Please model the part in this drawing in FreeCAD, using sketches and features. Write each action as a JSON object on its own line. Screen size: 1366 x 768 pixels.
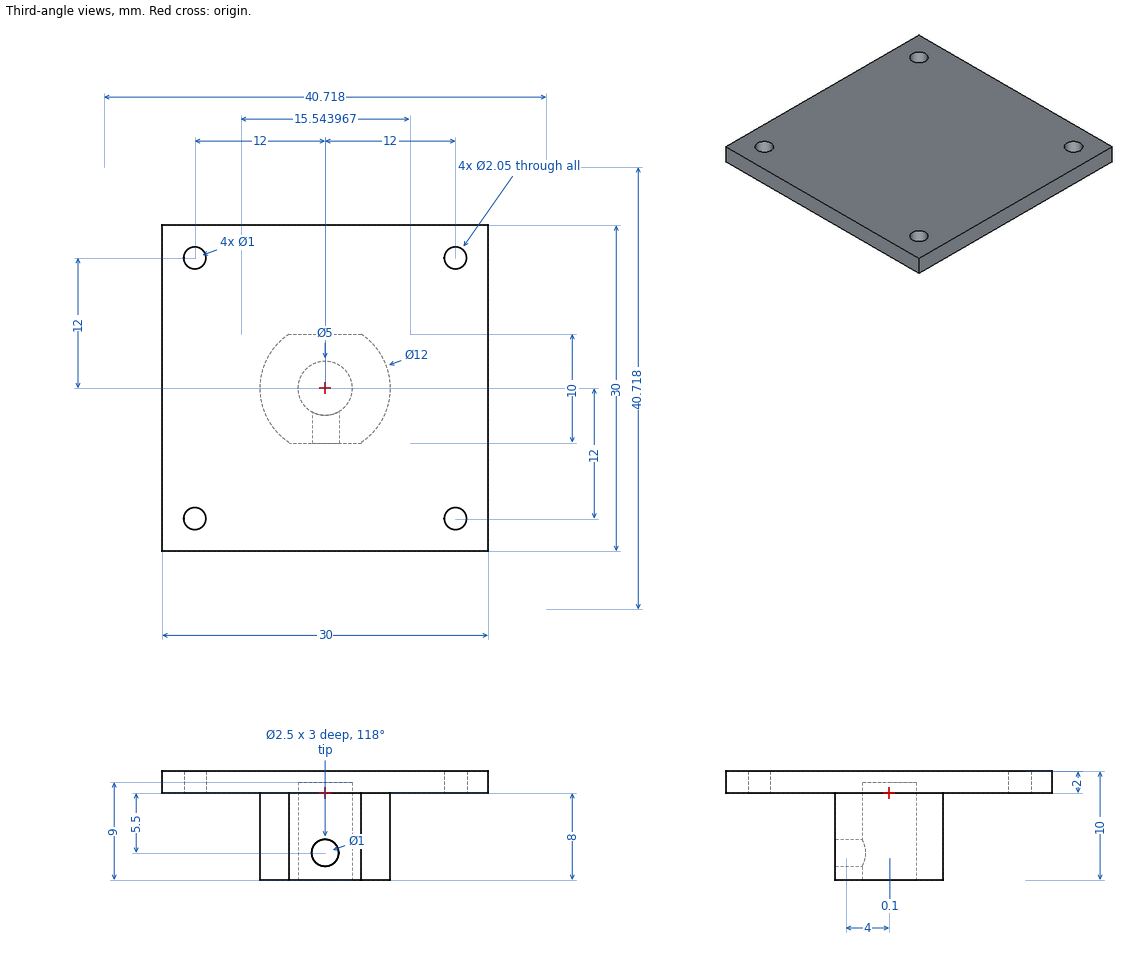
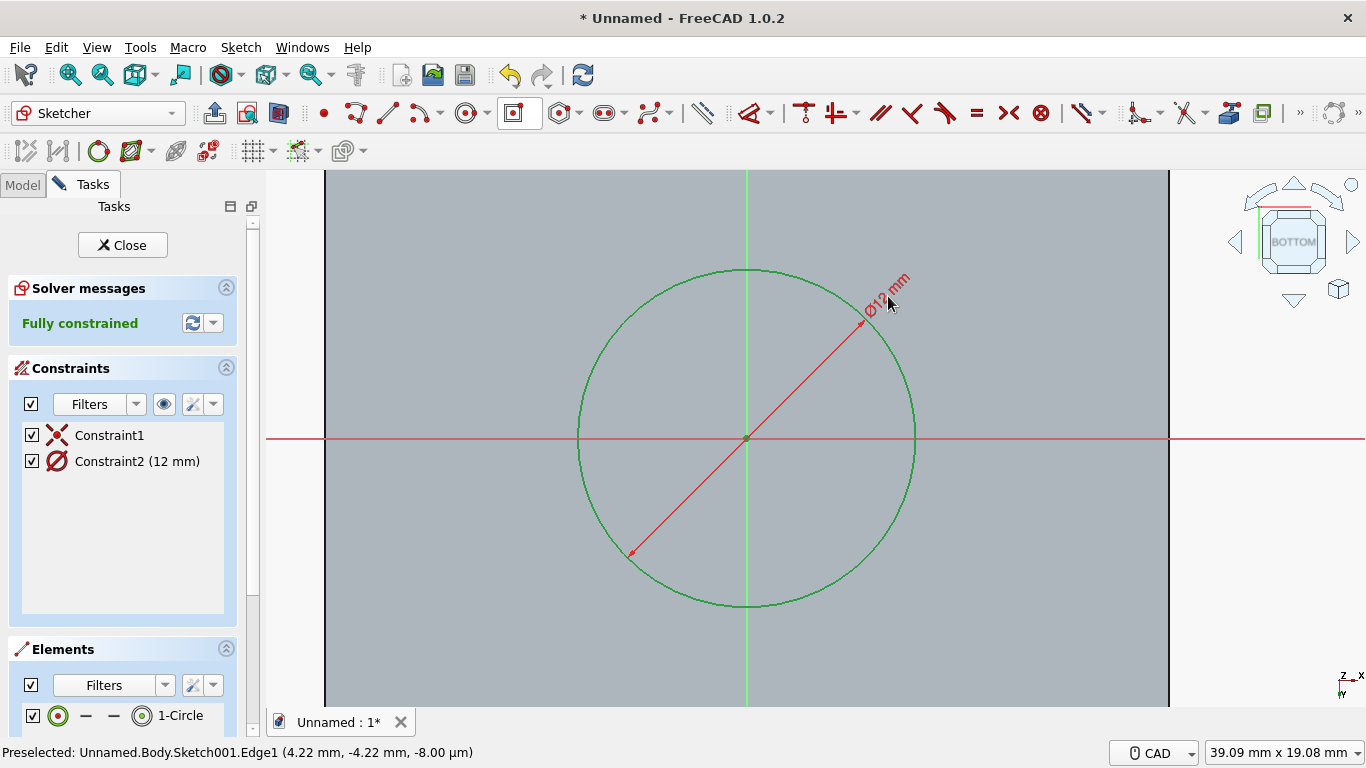
{"action": "left_click", "coordinate": [123, 245]}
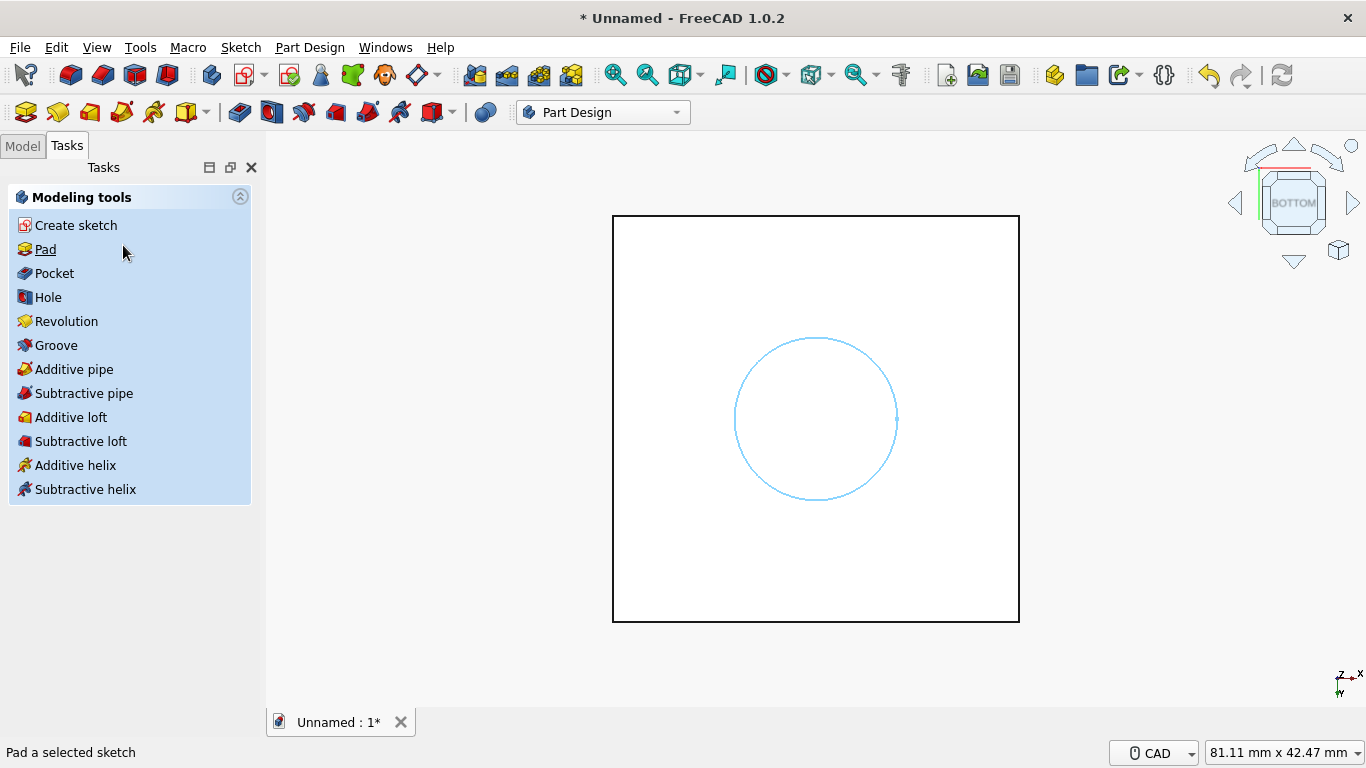
{"action": "left_click", "coordinate": [26, 112]}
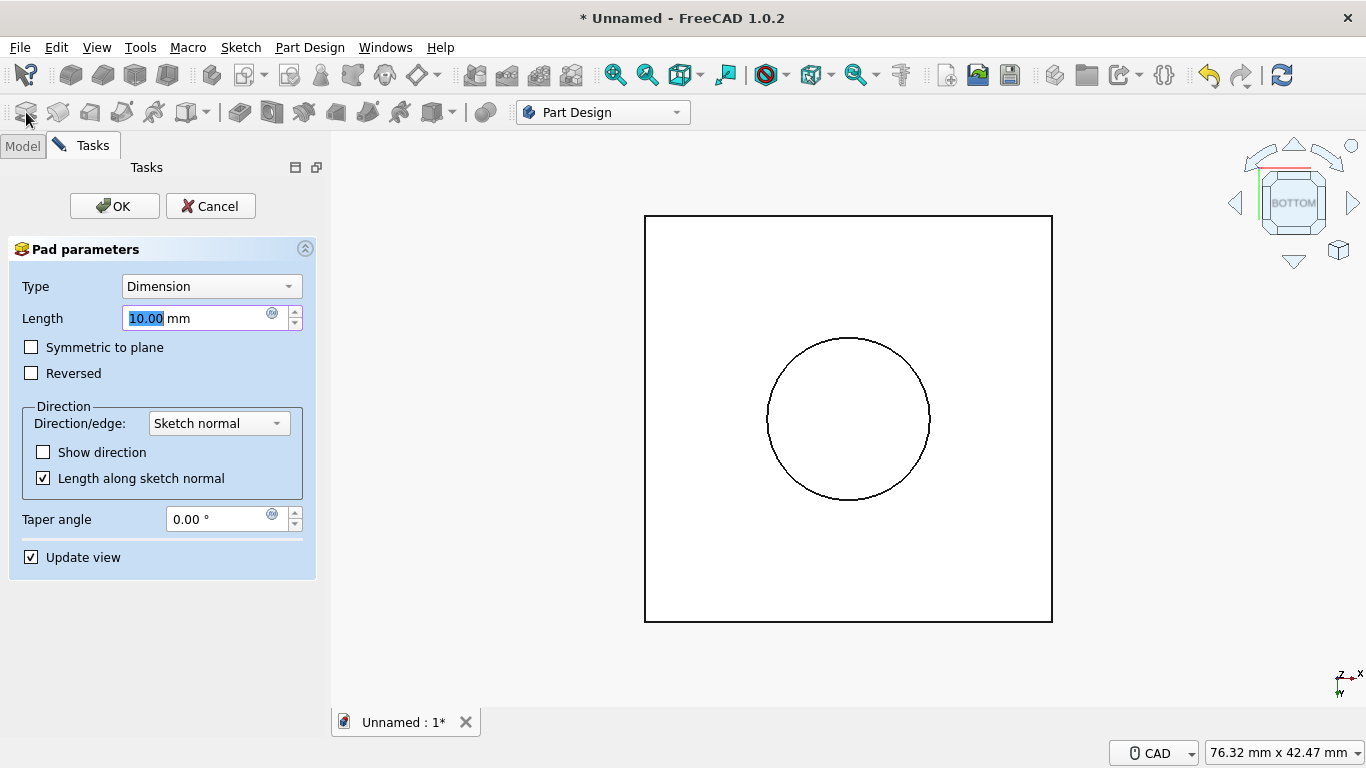
{"action": "type", "text": "8"}
{"action": "key", "text": "Tab"}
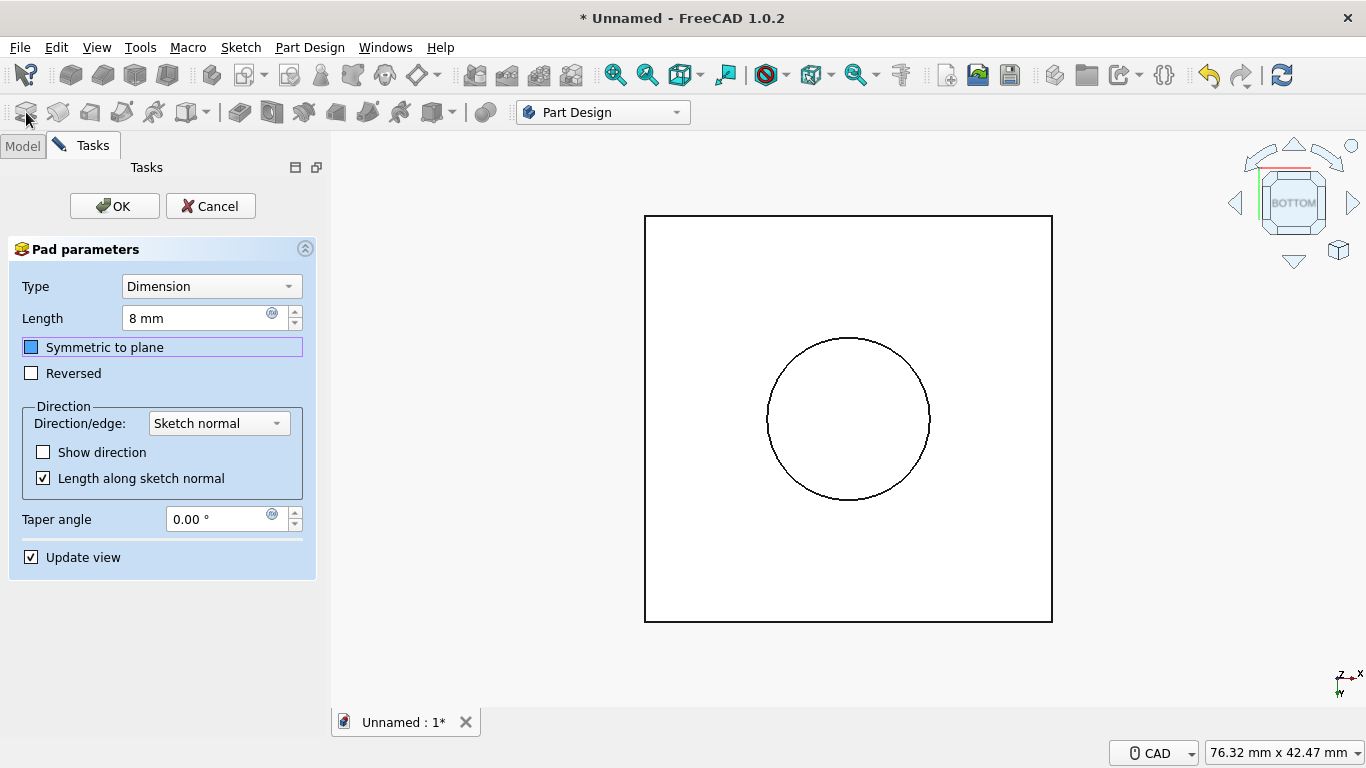
{"action": "left_click", "coordinate": [115, 206]}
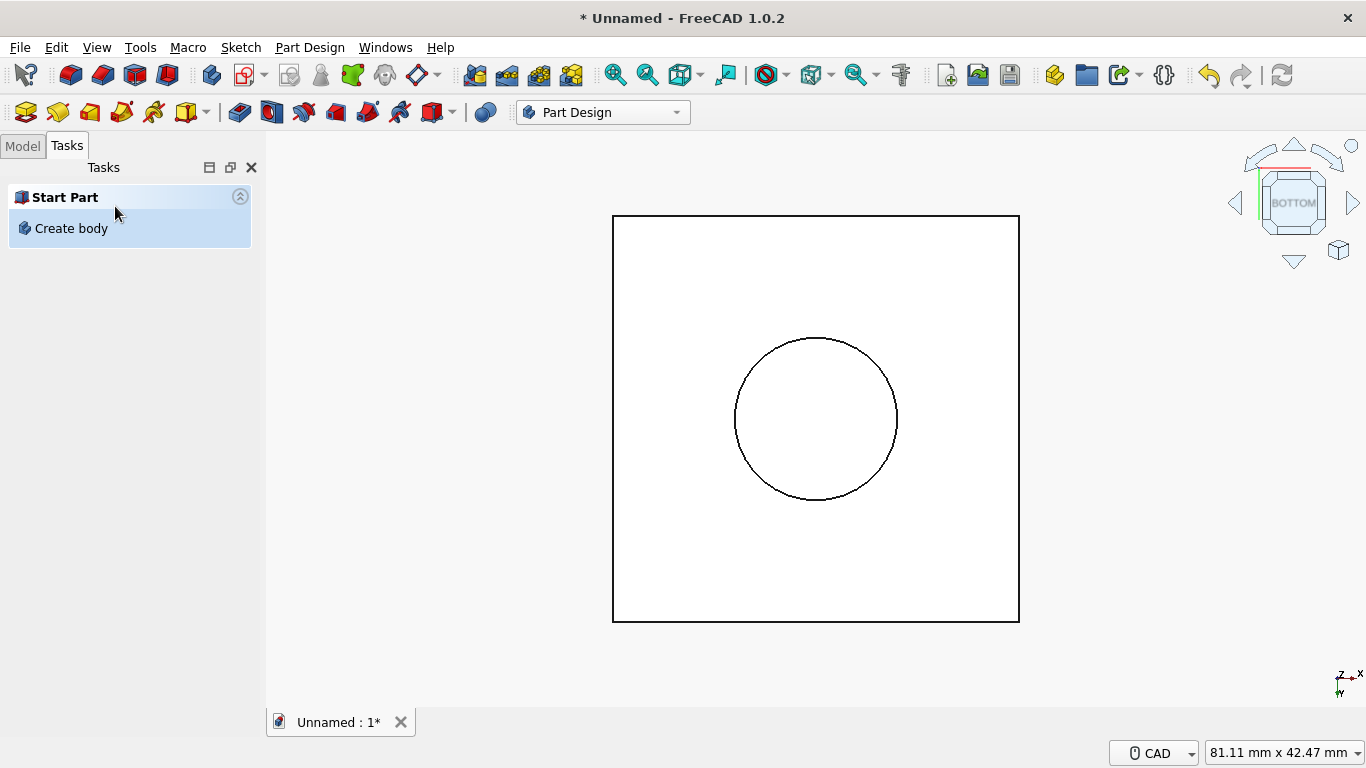
{"action": "key", "text": "0"}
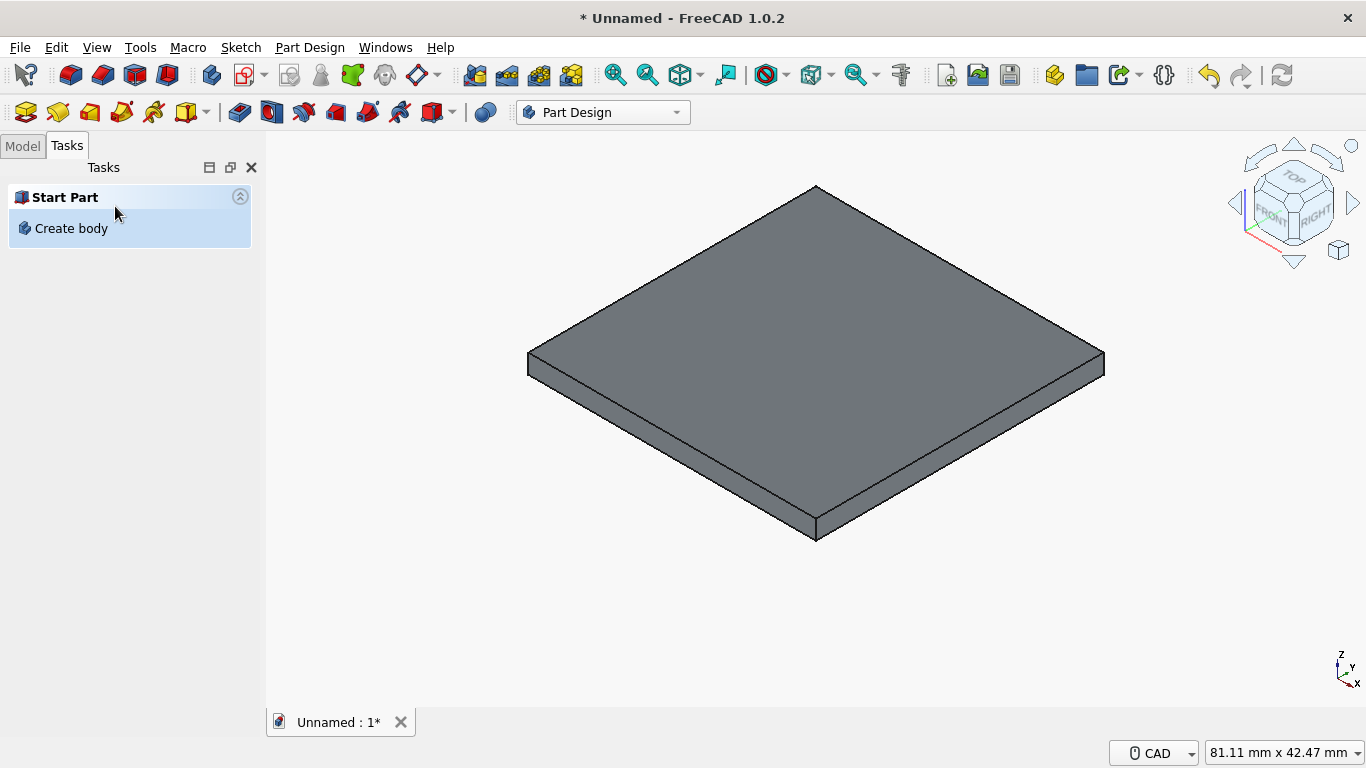
{"action": "left_click", "coordinate": [816, 352]}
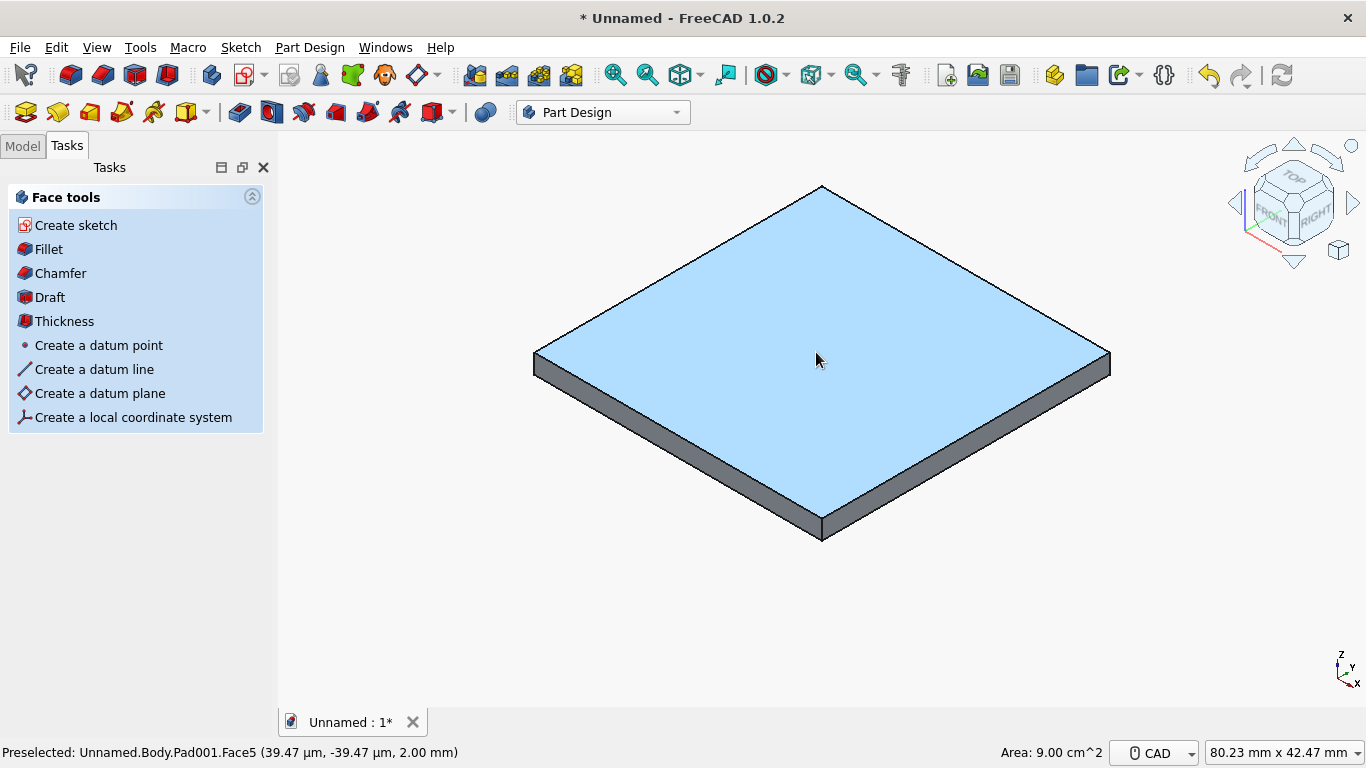
{"action": "left_click", "coordinate": [244, 76]}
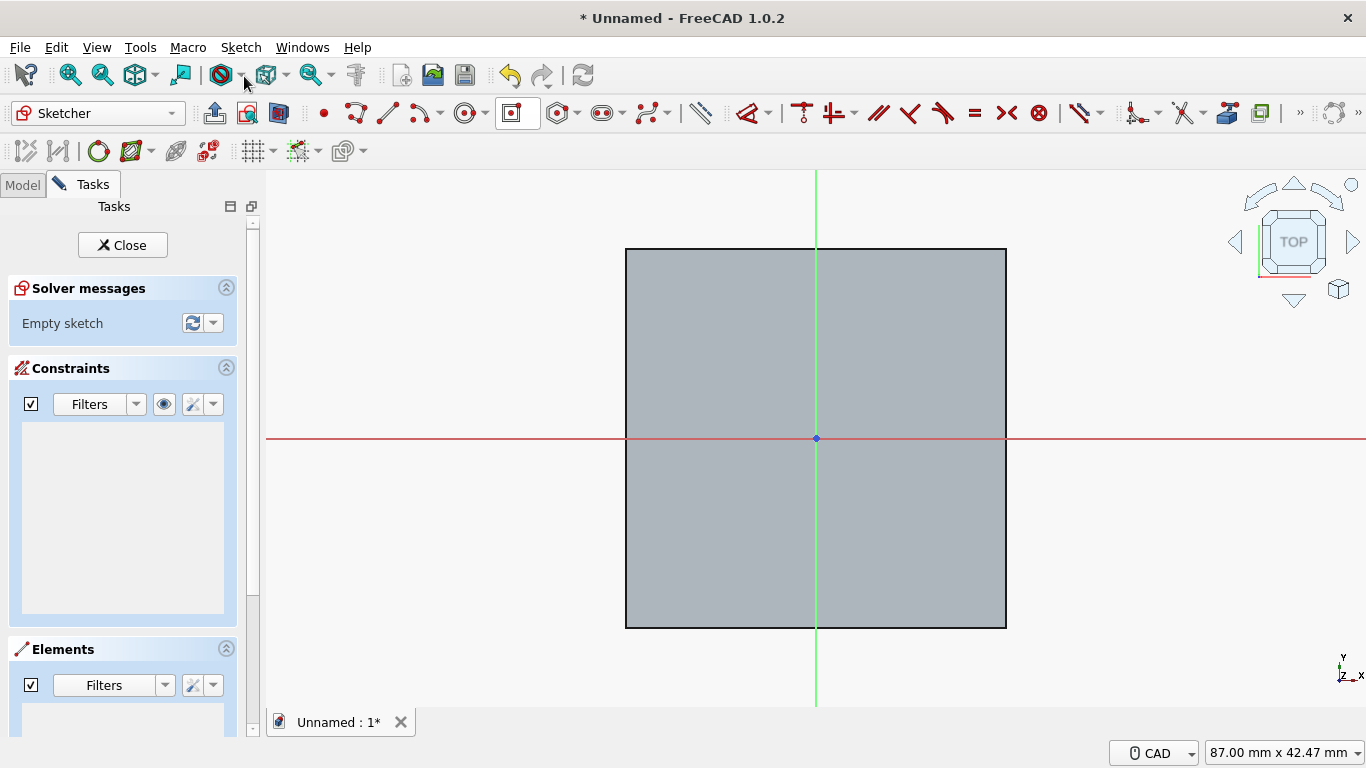
{"action": "key", "text": "g c"}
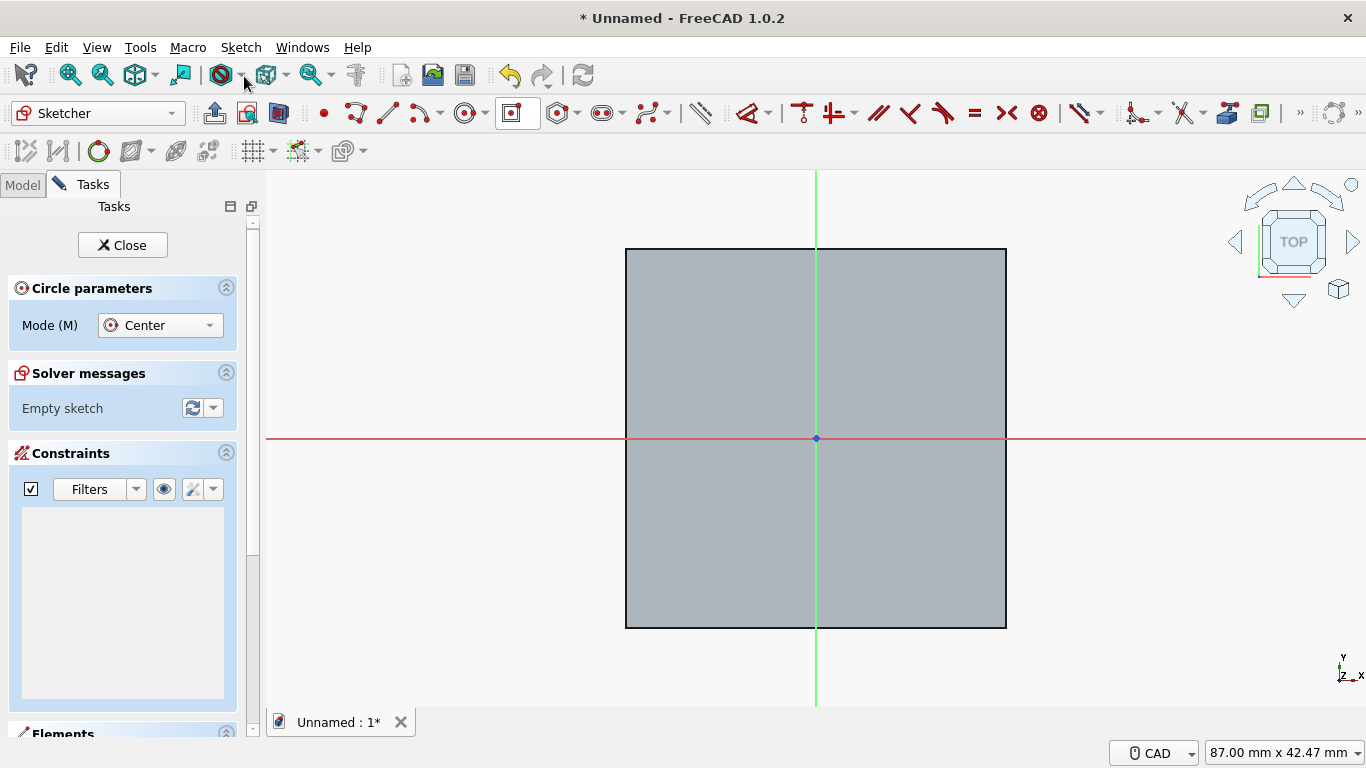
{"action": "scroll", "coordinate": [664, 287], "scroll_direction": "up", "scroll_amount": 7}